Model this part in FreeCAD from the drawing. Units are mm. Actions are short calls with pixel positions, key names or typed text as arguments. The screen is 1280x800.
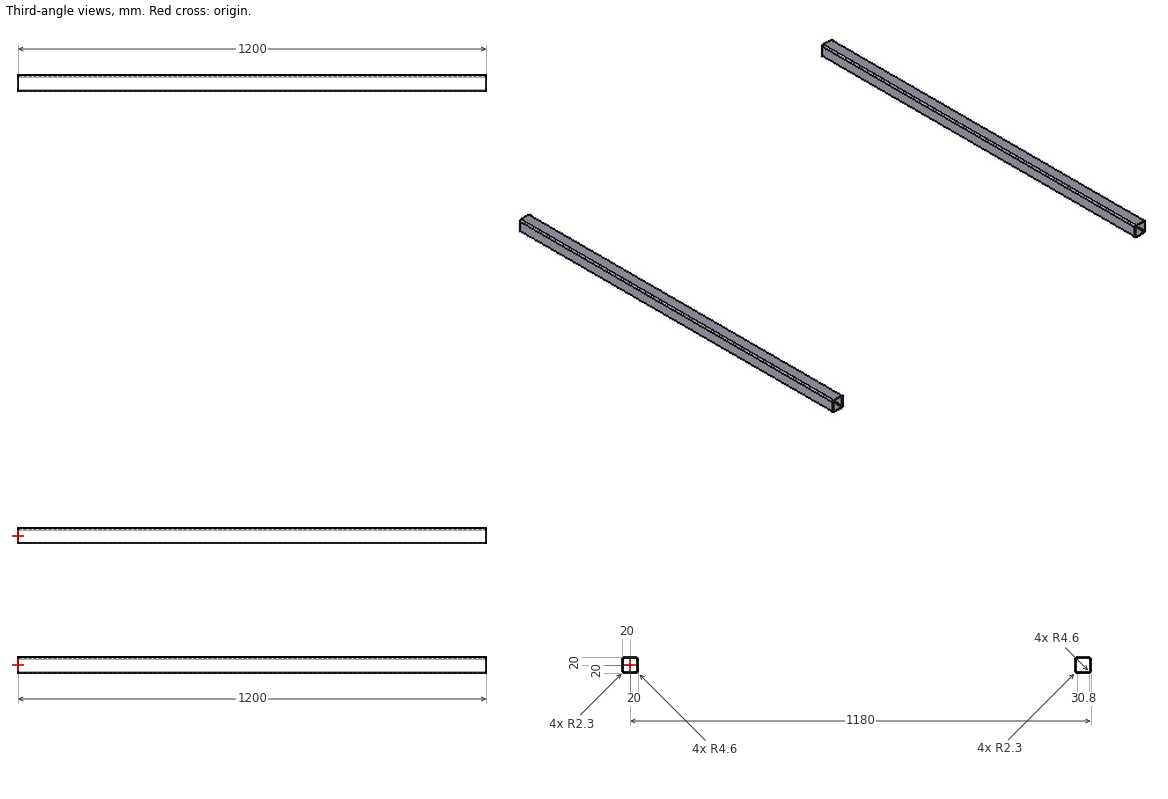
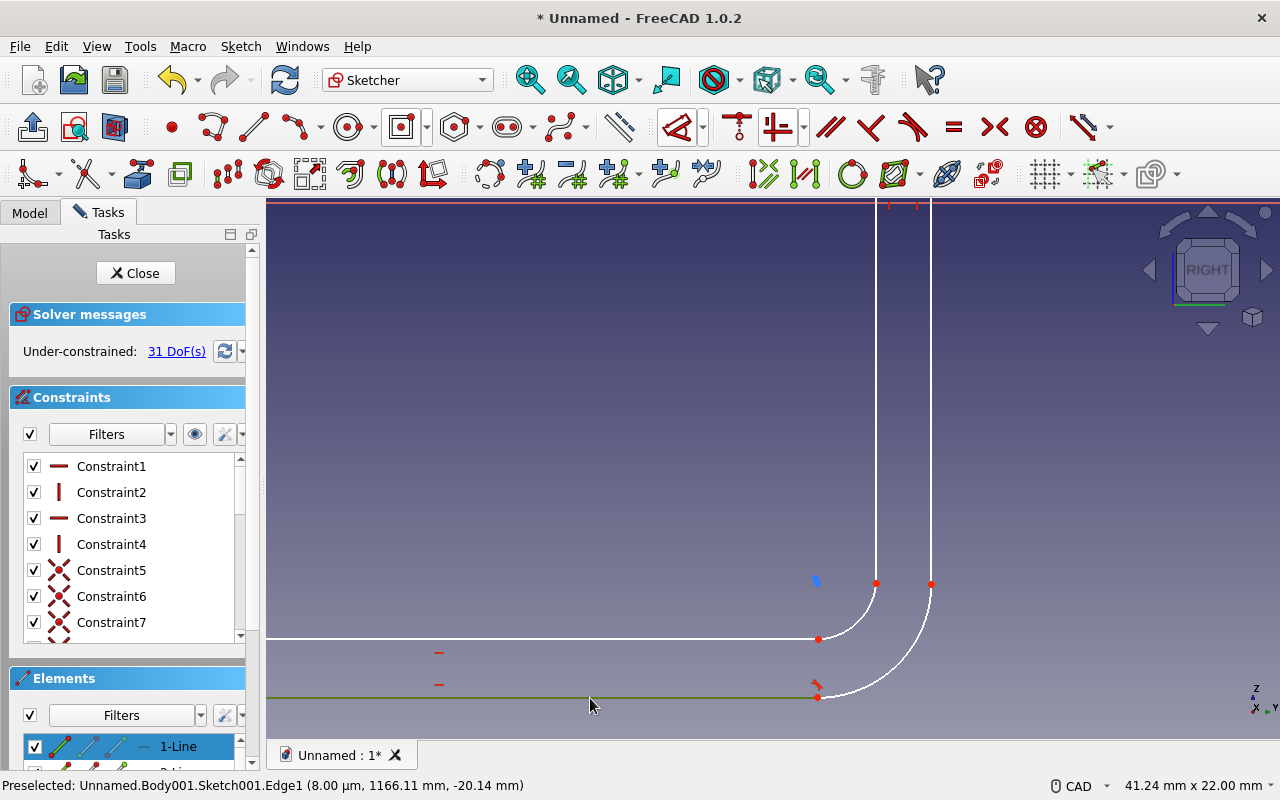
scroll(859, 623, down, 5)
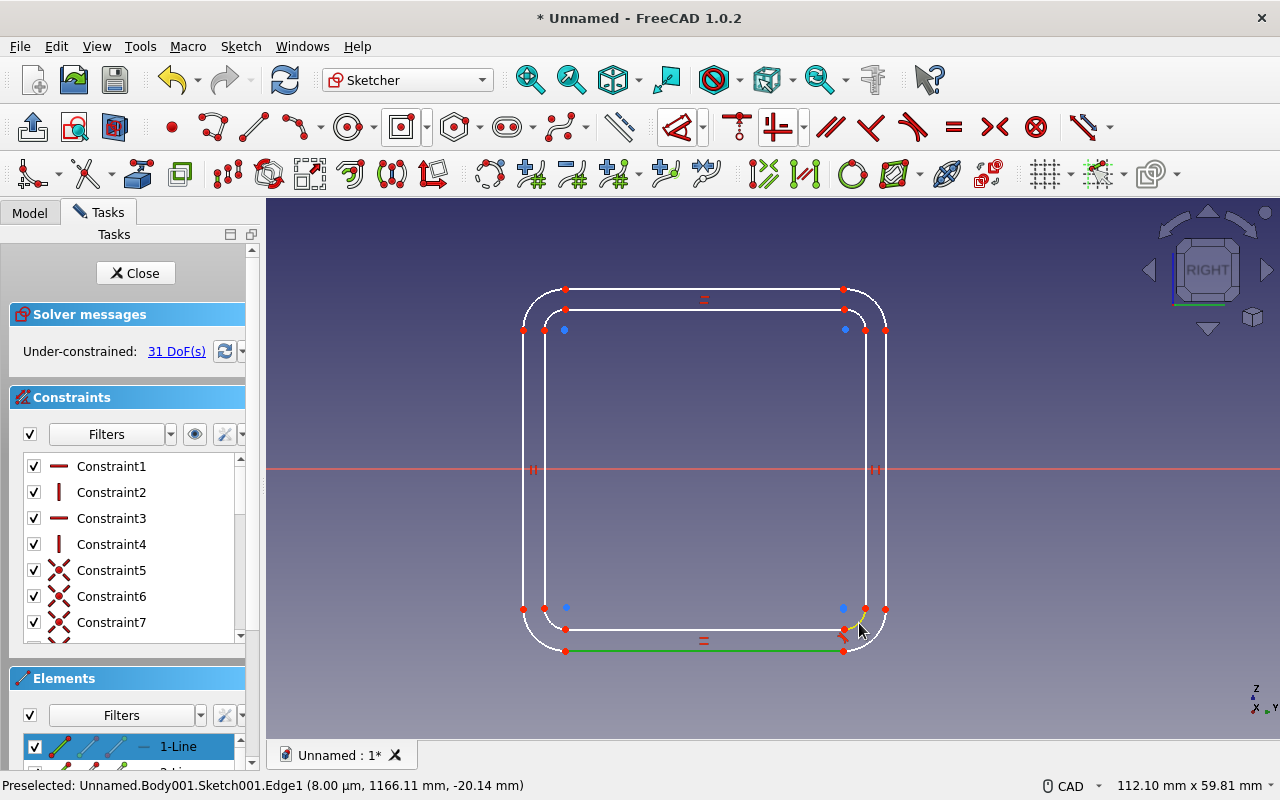
click(528, 628)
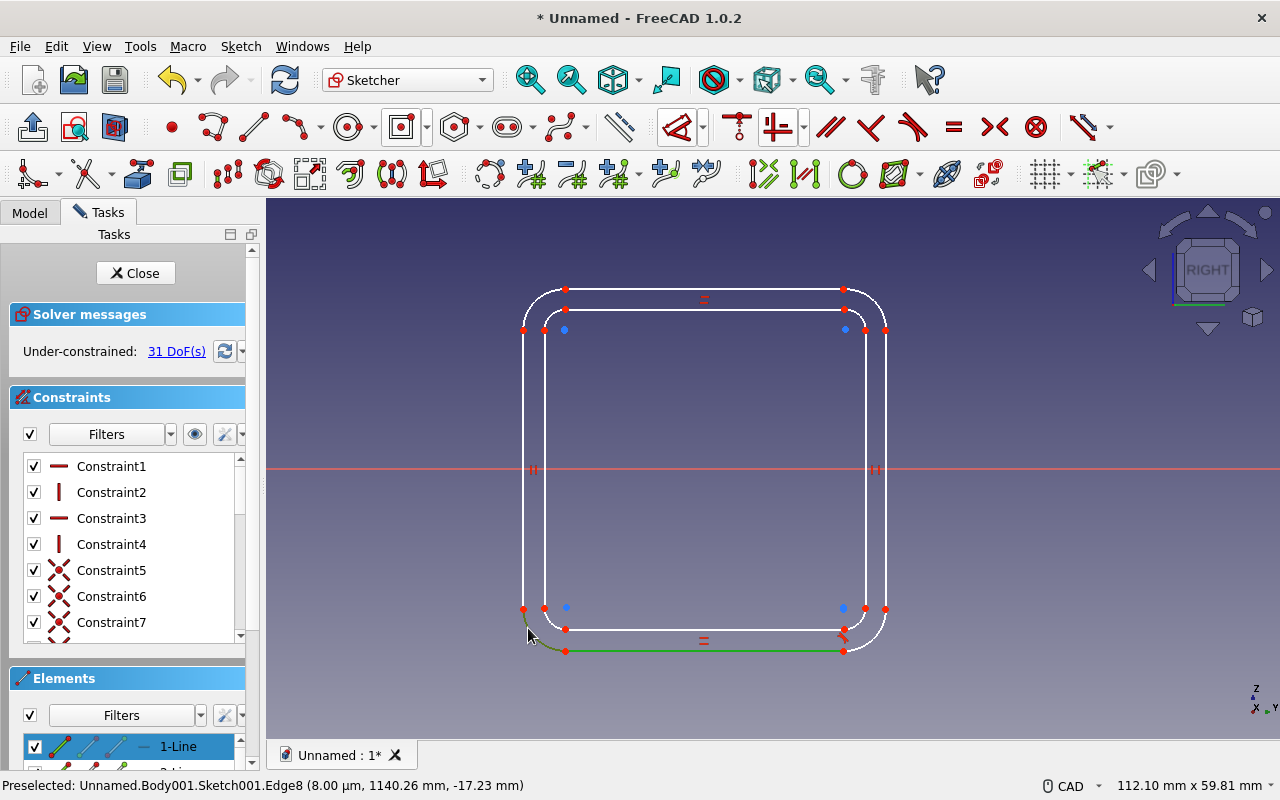
click(913, 128)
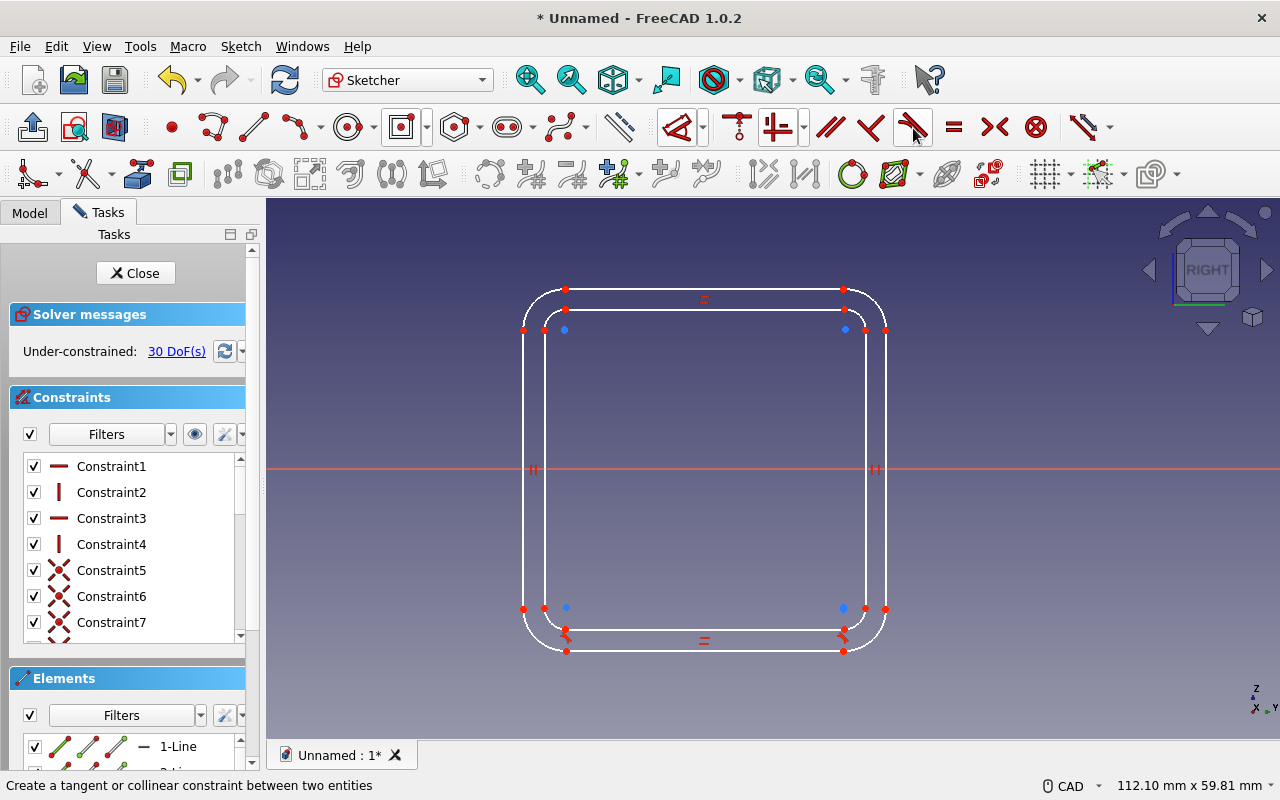
click(886, 526)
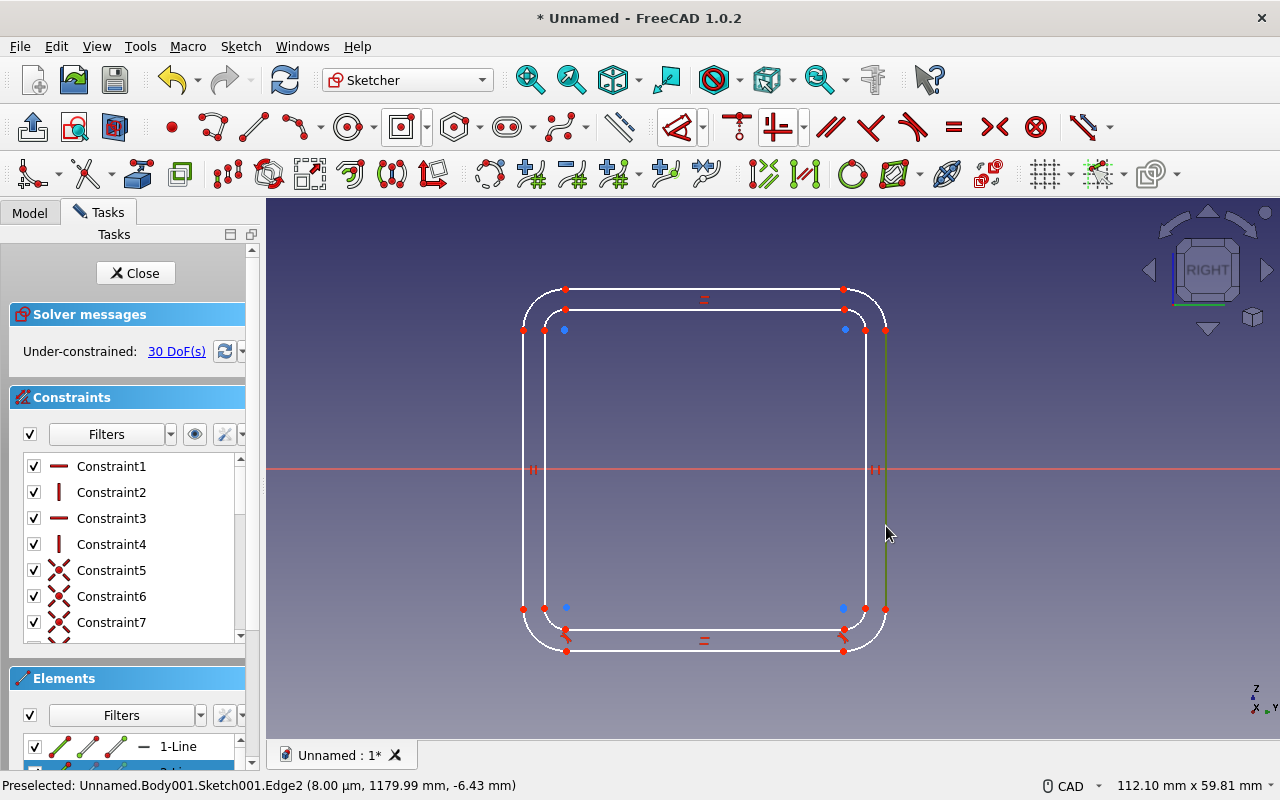
click(863, 647)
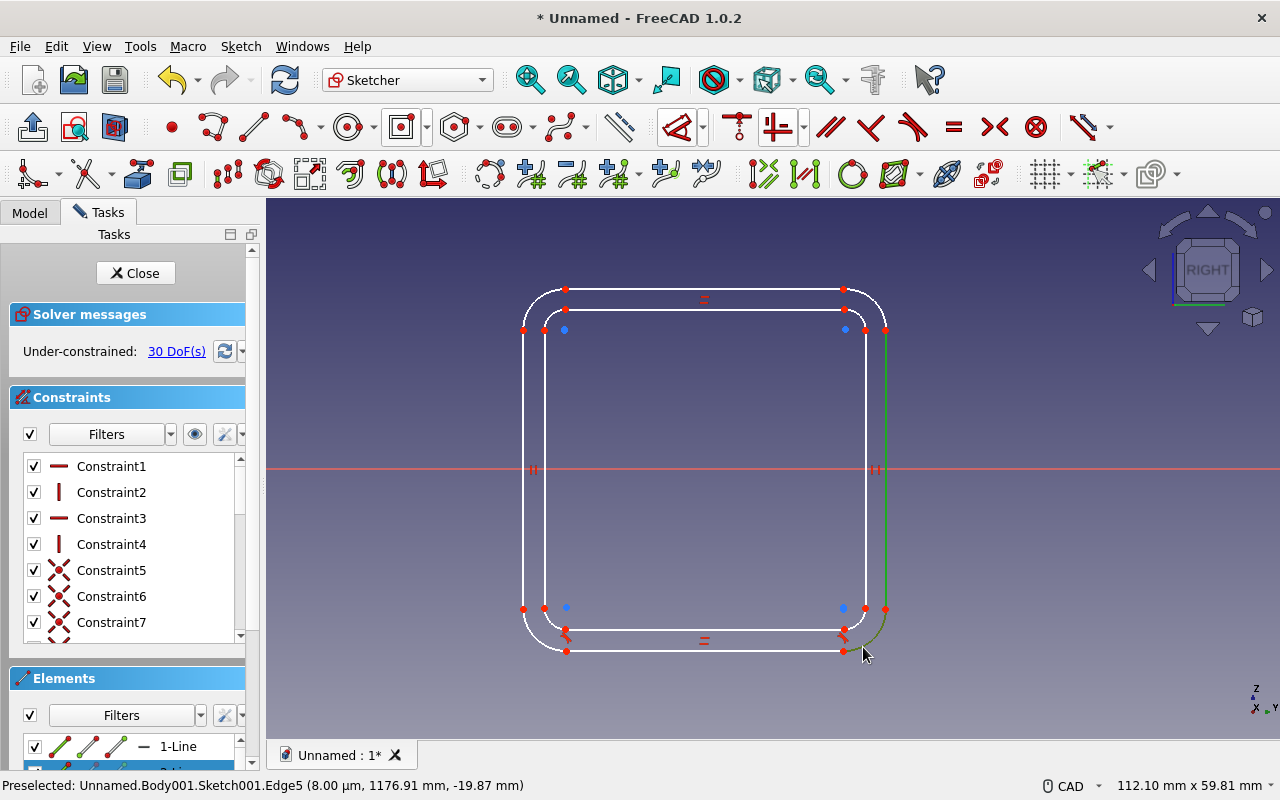
key(t)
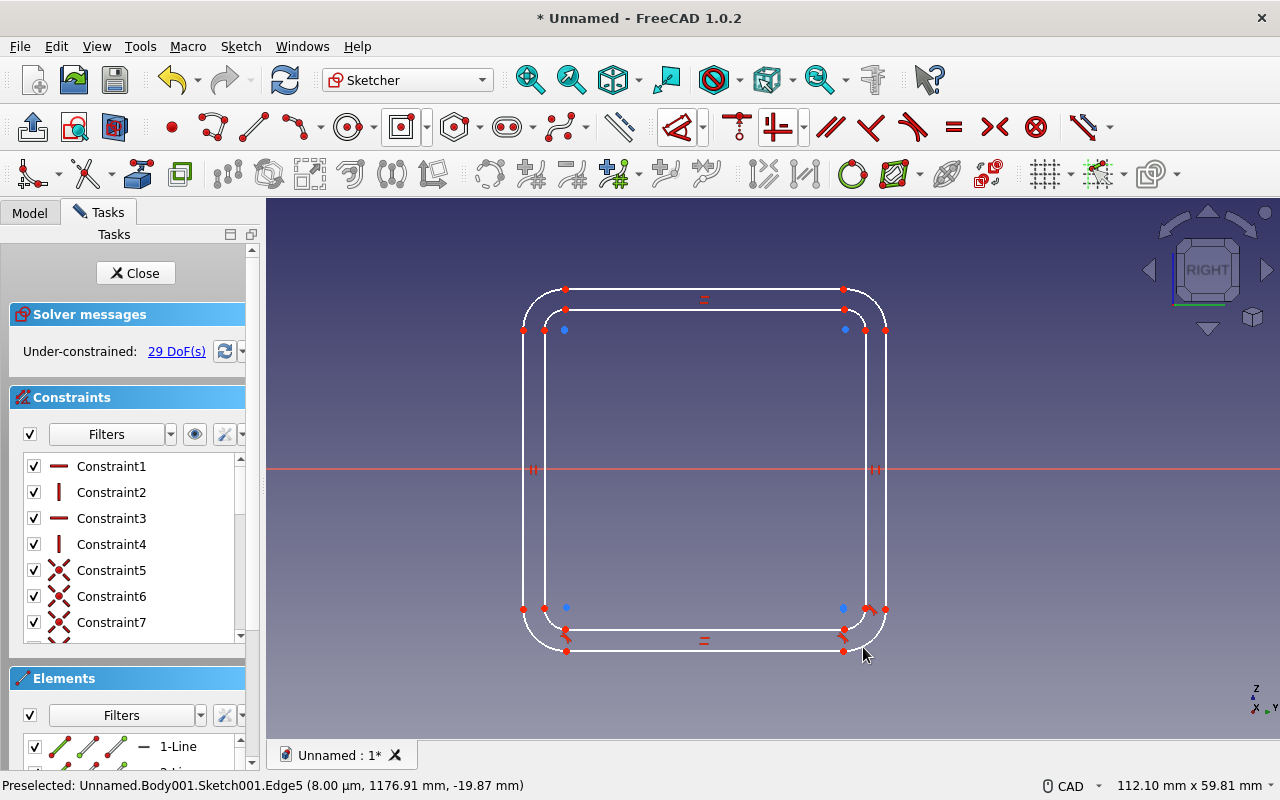
click(886, 525)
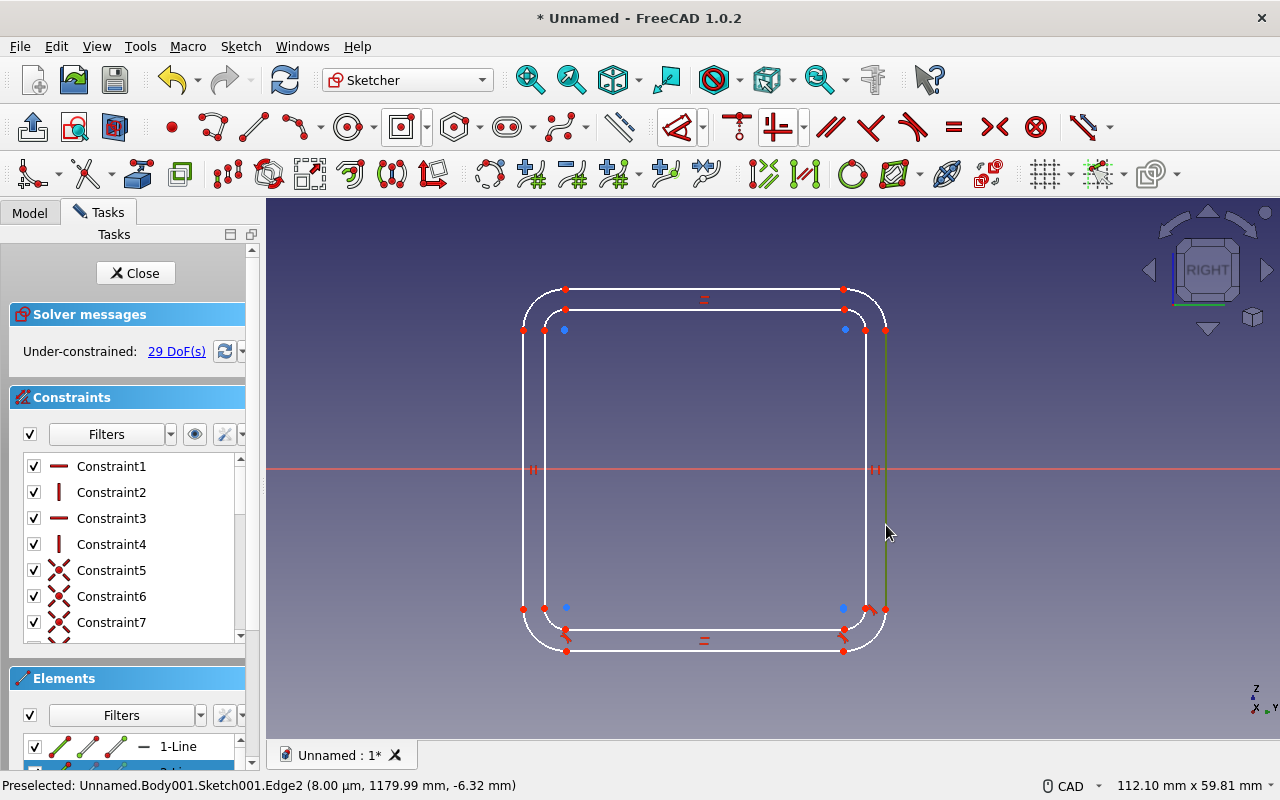
click(882, 311)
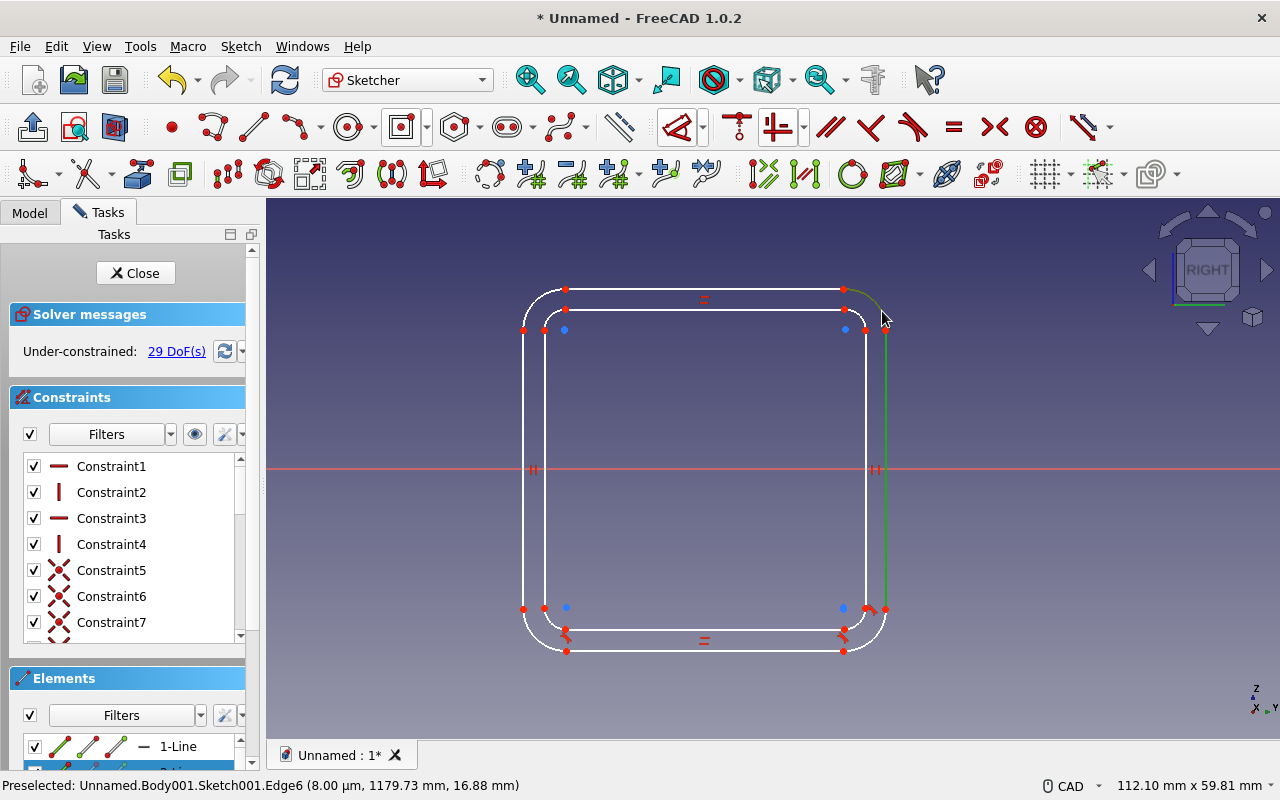
key(t)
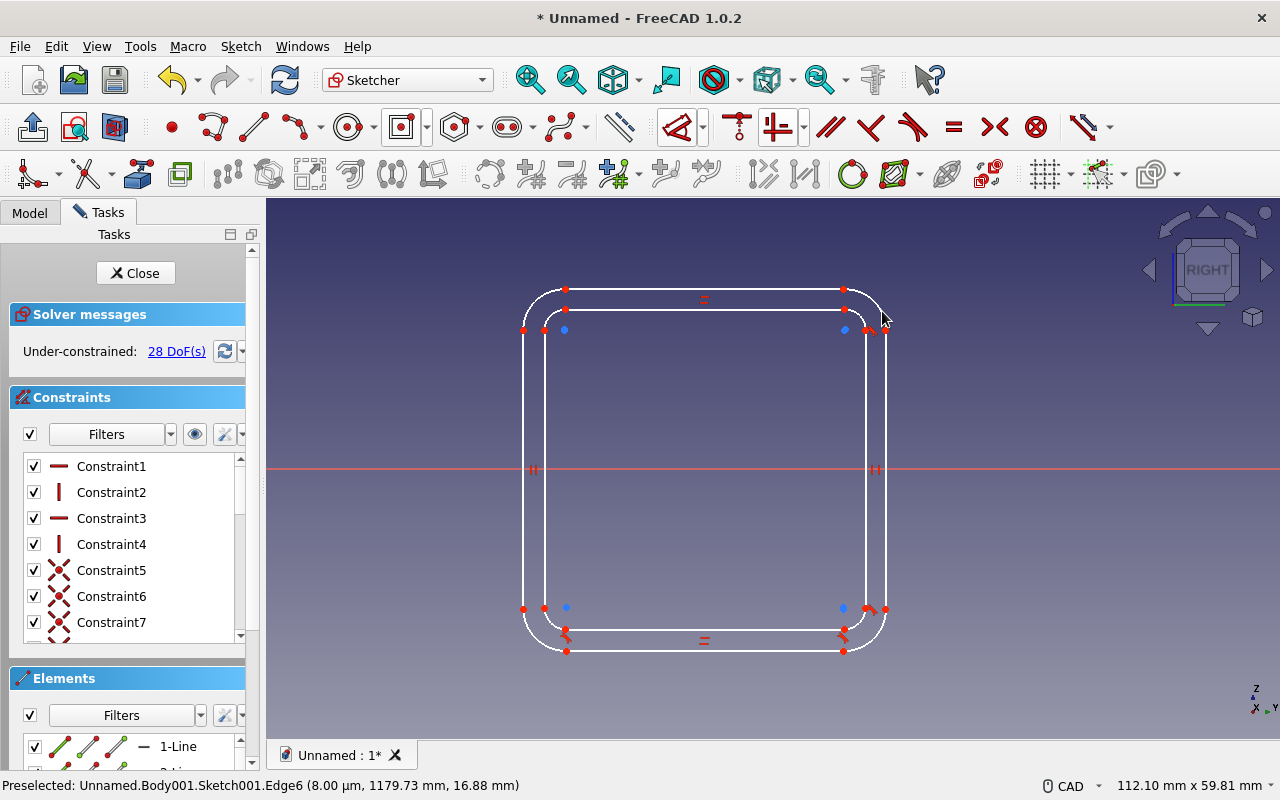
click(761, 289)